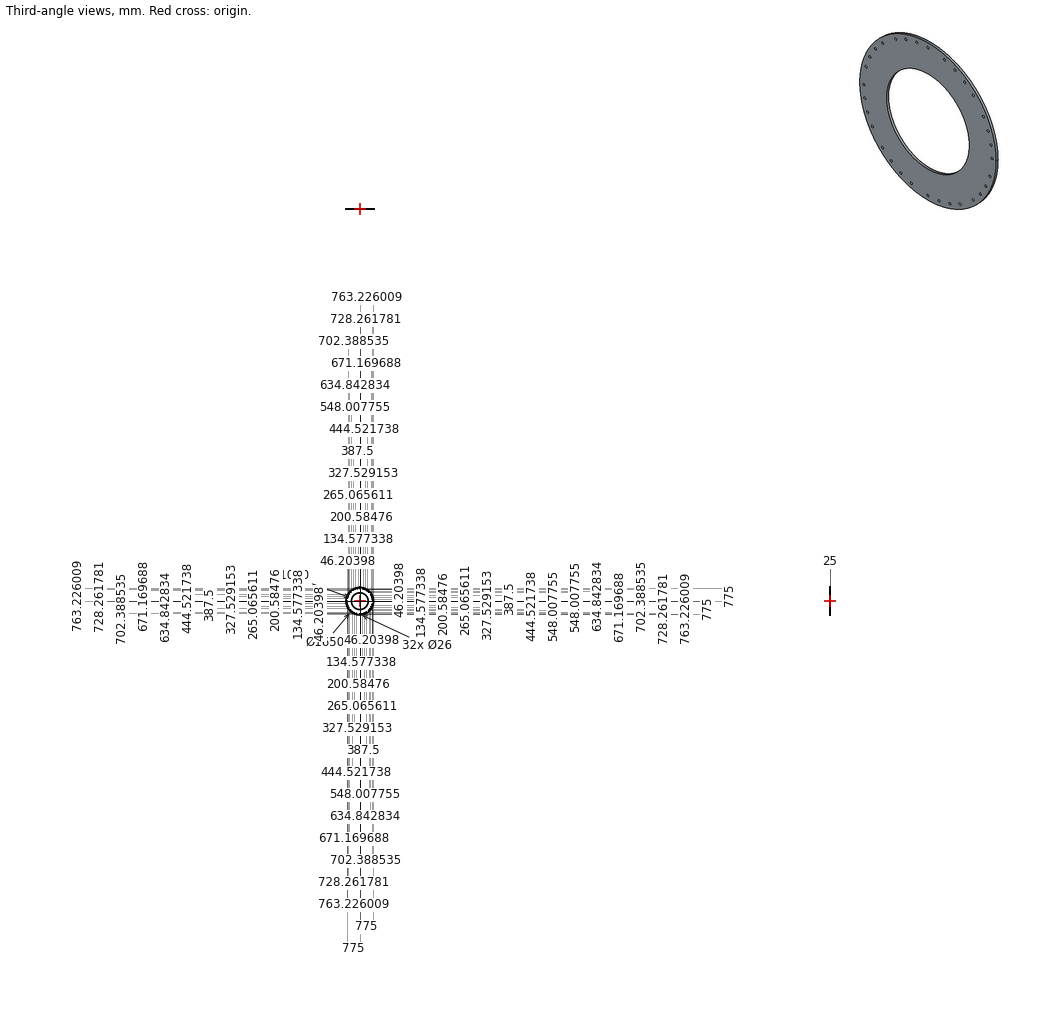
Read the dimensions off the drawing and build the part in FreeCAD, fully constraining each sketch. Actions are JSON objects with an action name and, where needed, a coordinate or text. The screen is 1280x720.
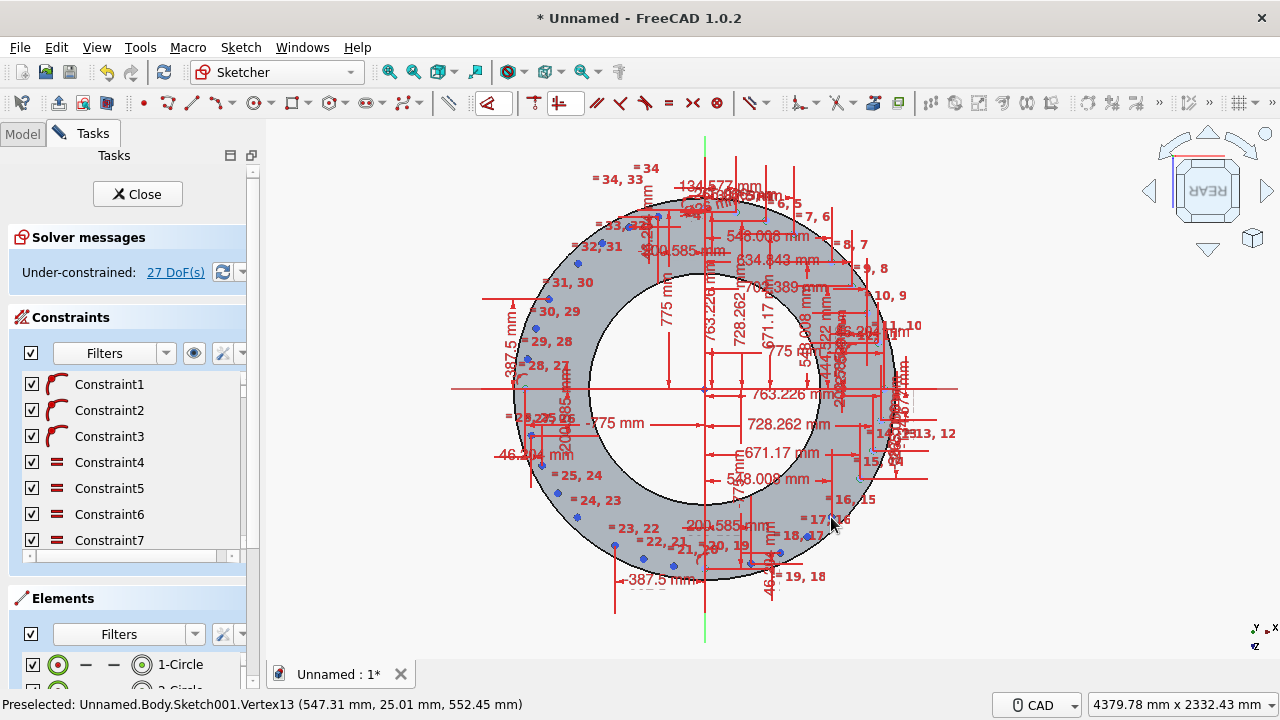
{"action": "left_click", "coordinate": [832, 517]}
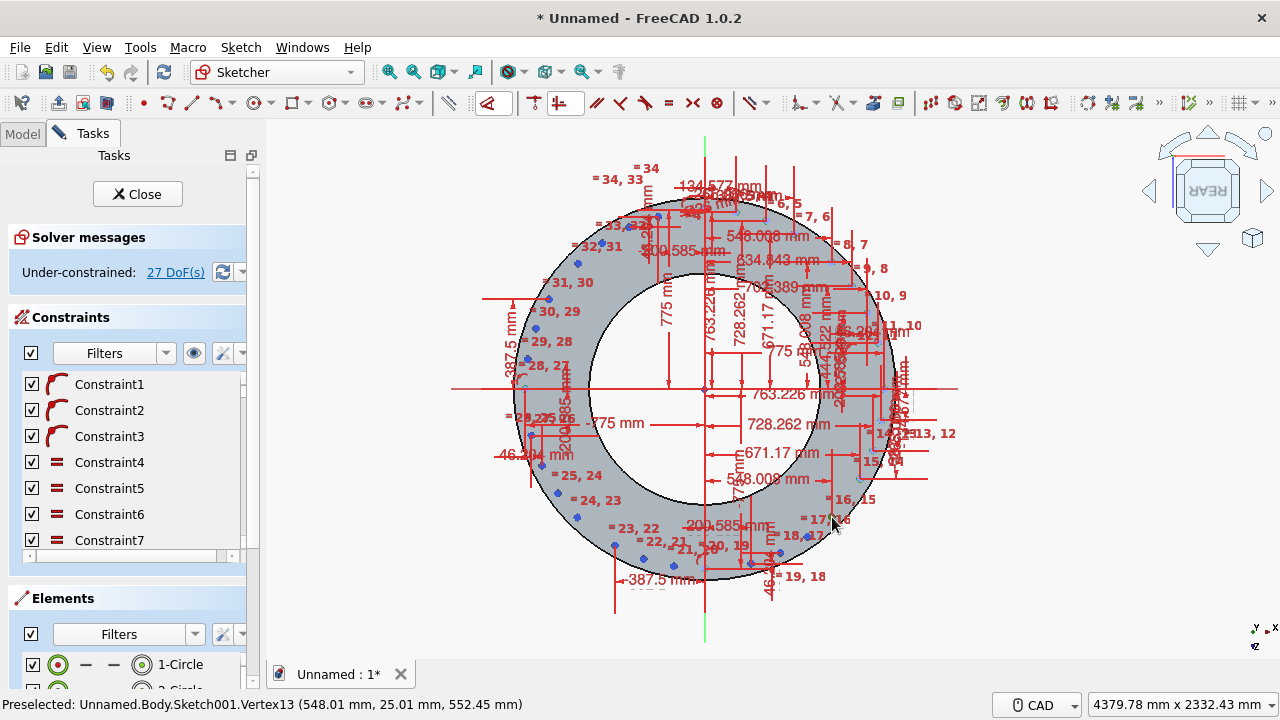
{"action": "key", "text": "i"}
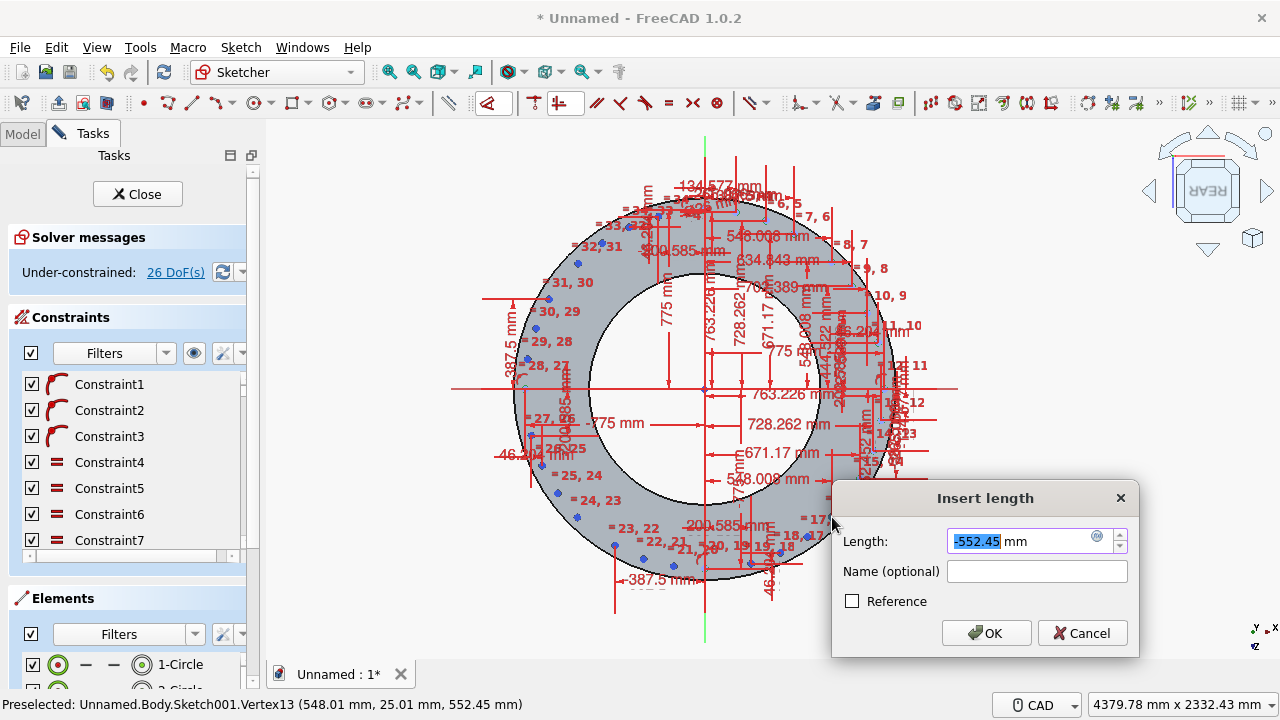
{"action": "type", "text": "-548.007755"}
{"action": "key", "text": "Return"}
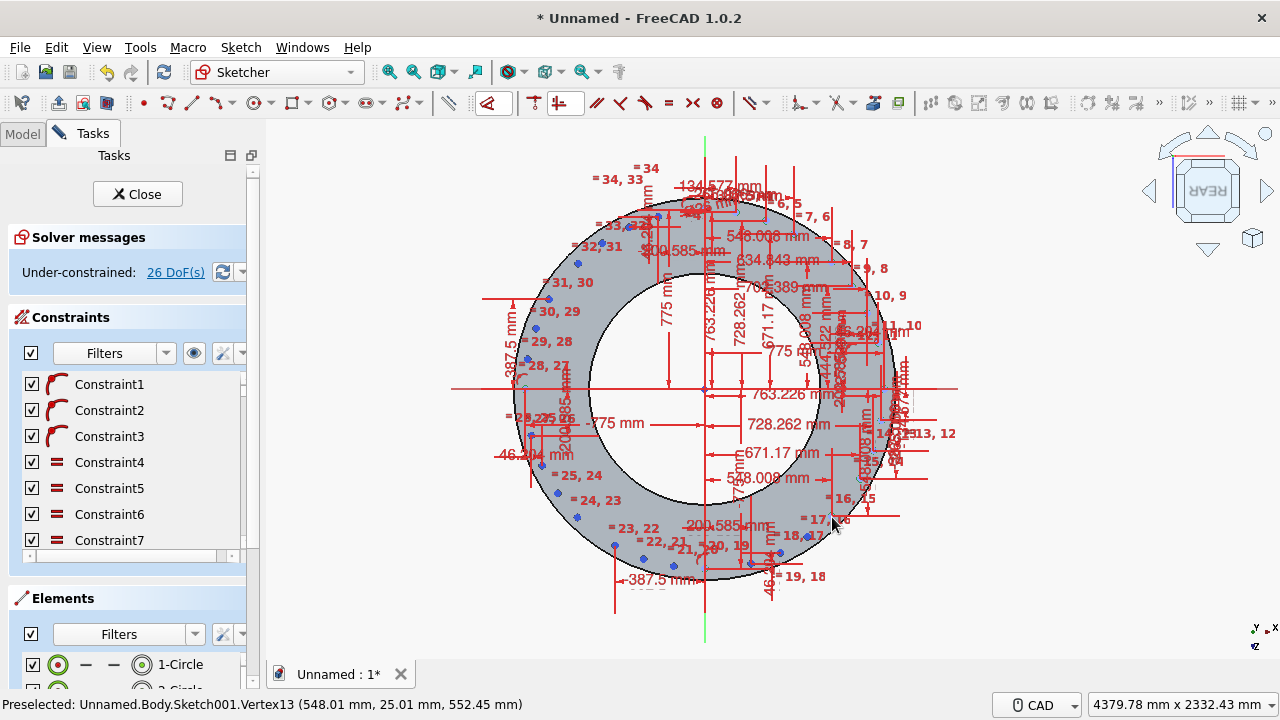
{"action": "left_click", "coordinate": [807, 537]}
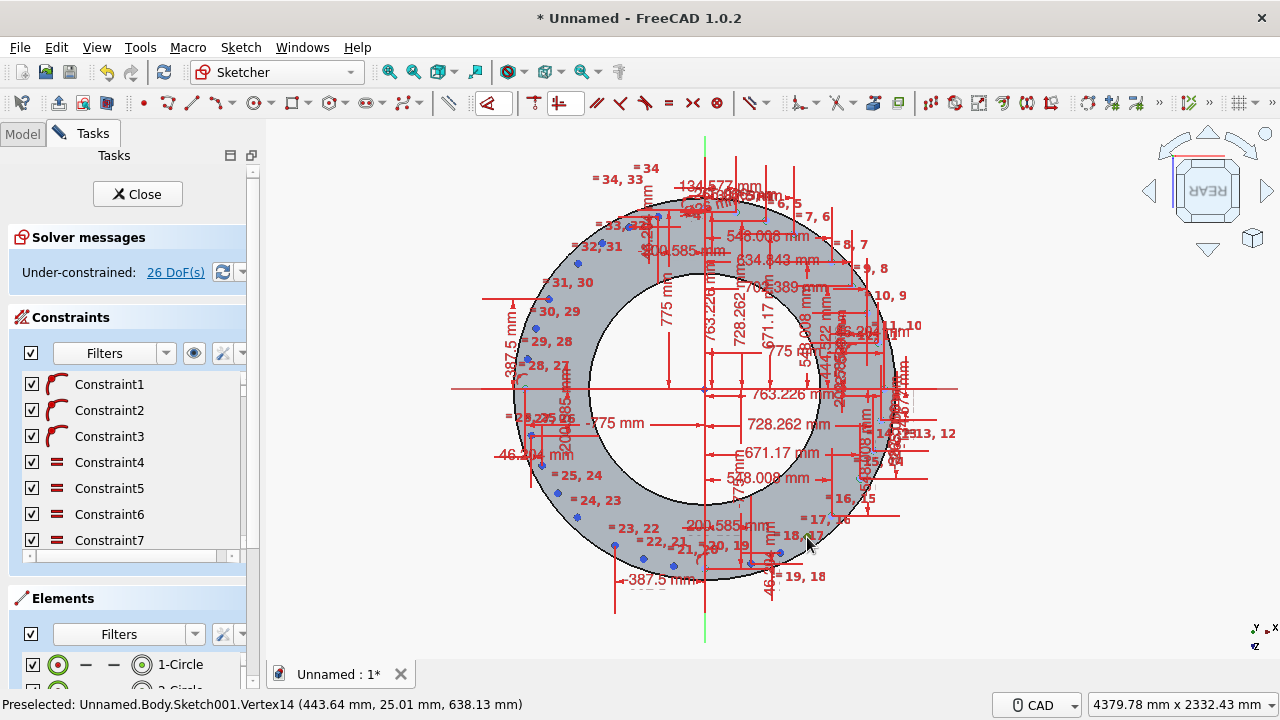
{"action": "key", "text": "l"}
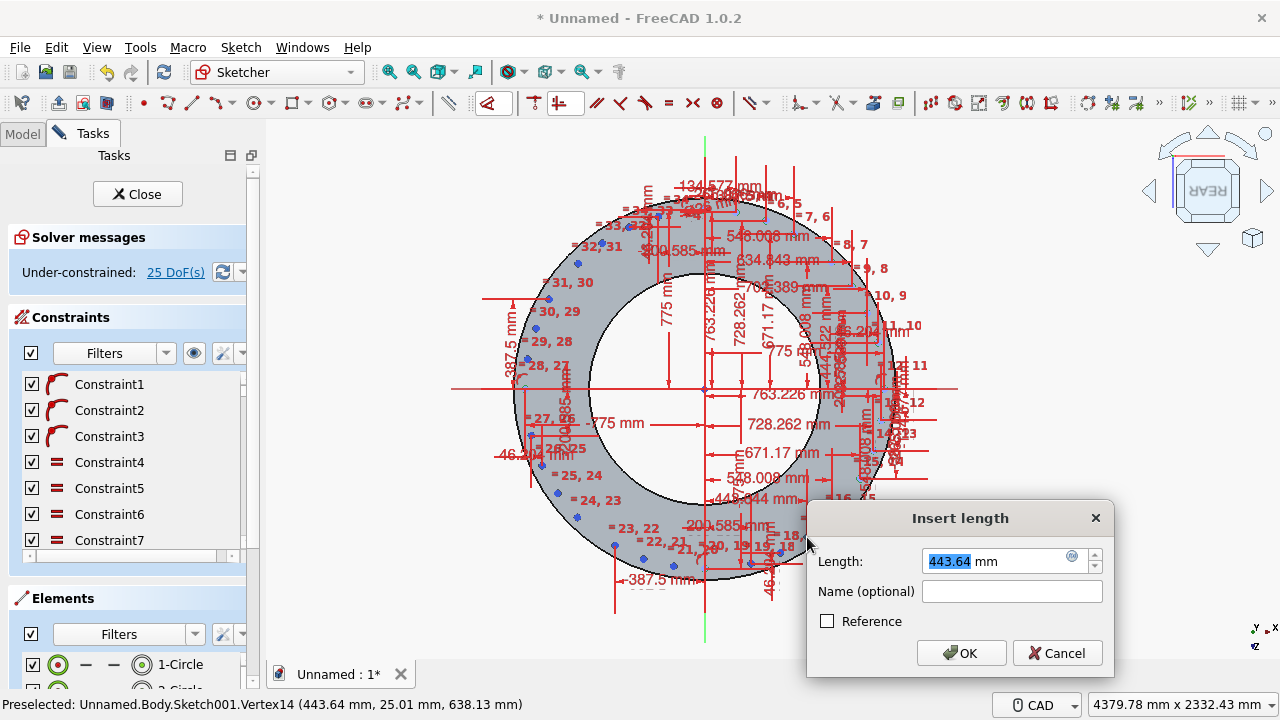
{"action": "type", "text": "444.521738"}
{"action": "key", "text": "Return"}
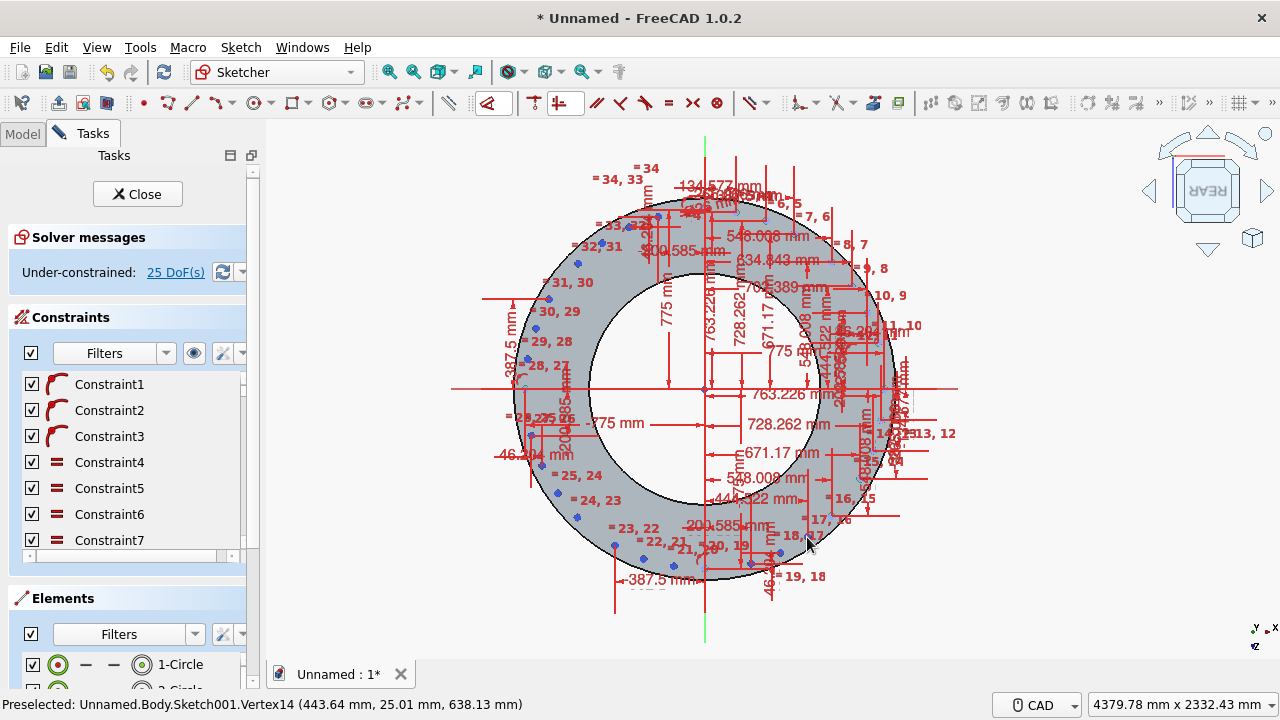
{"action": "left_click", "coordinate": [808, 537]}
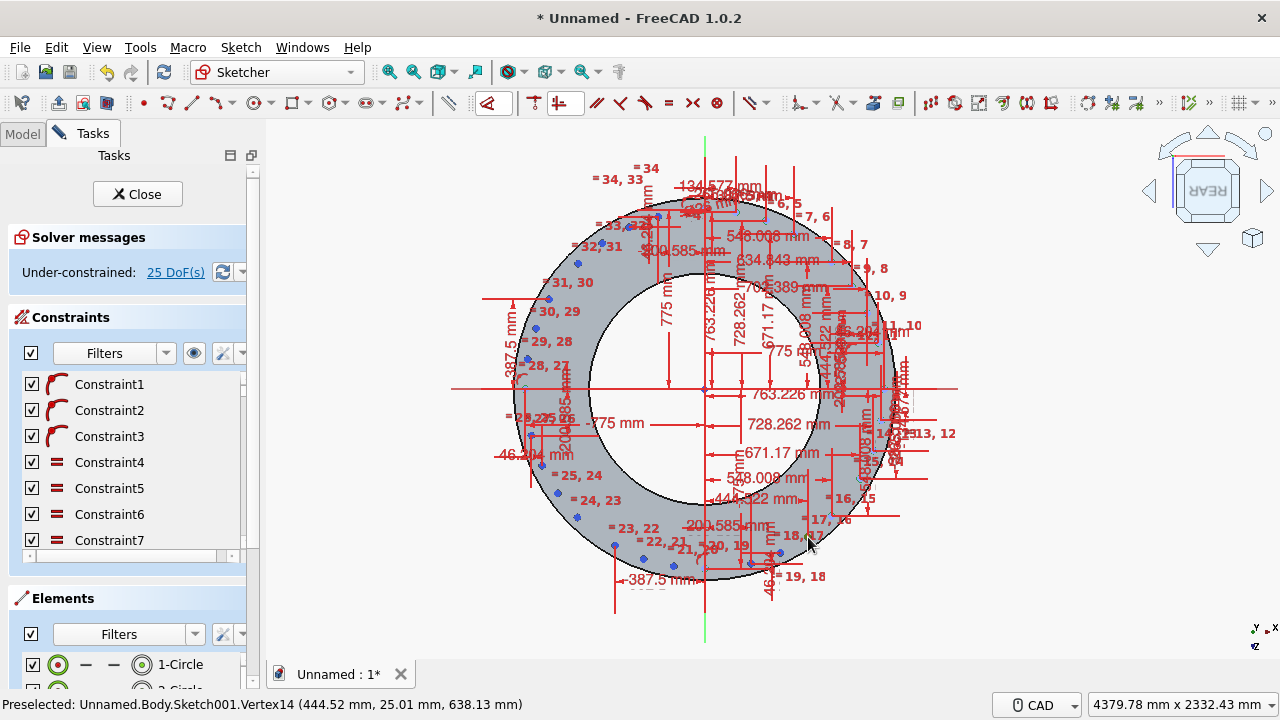
{"action": "key", "text": "i"}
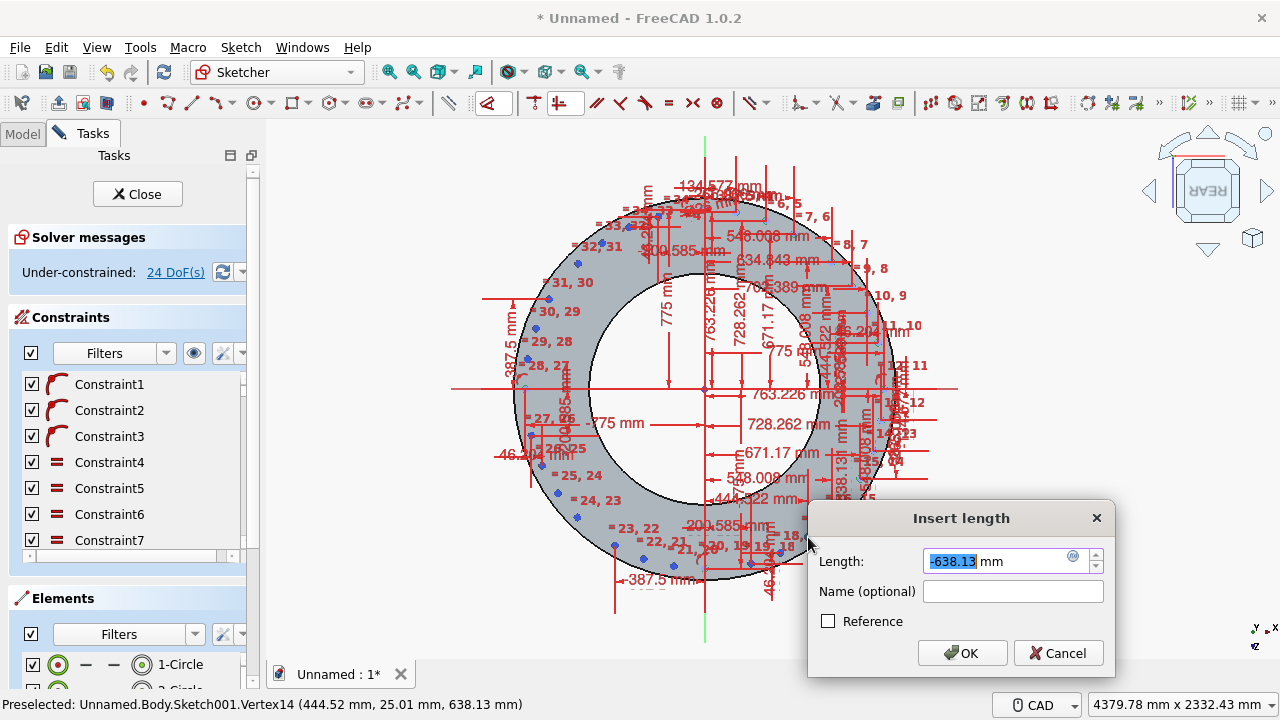
{"action": "type", "text": "-634.842834"}
{"action": "key", "text": "Return"}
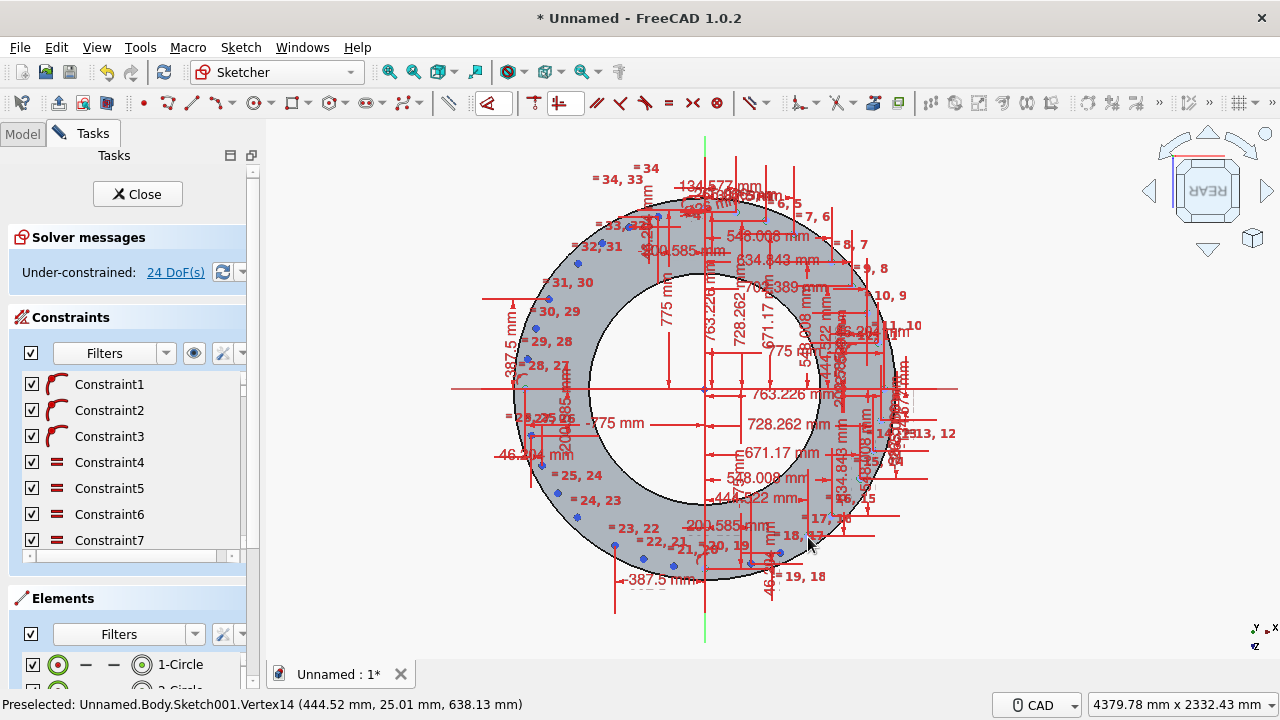
{"action": "left_click", "coordinate": [780, 553]}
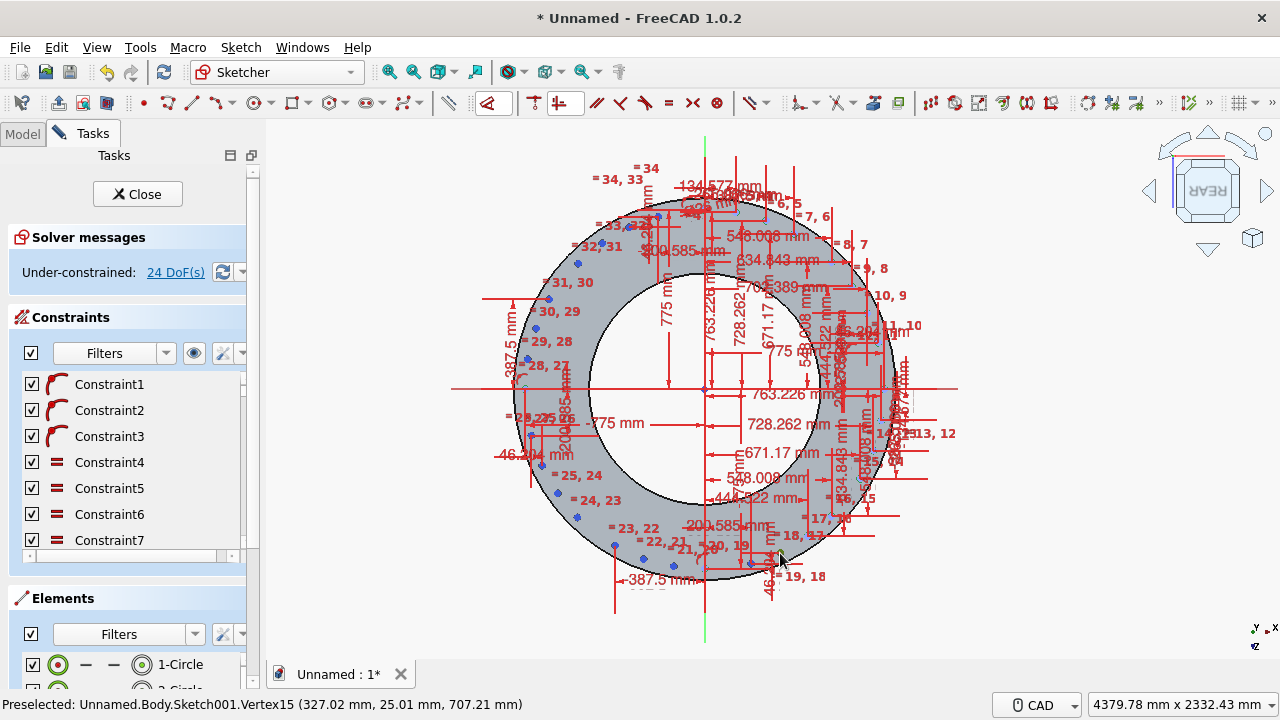
{"action": "key", "text": "l"}